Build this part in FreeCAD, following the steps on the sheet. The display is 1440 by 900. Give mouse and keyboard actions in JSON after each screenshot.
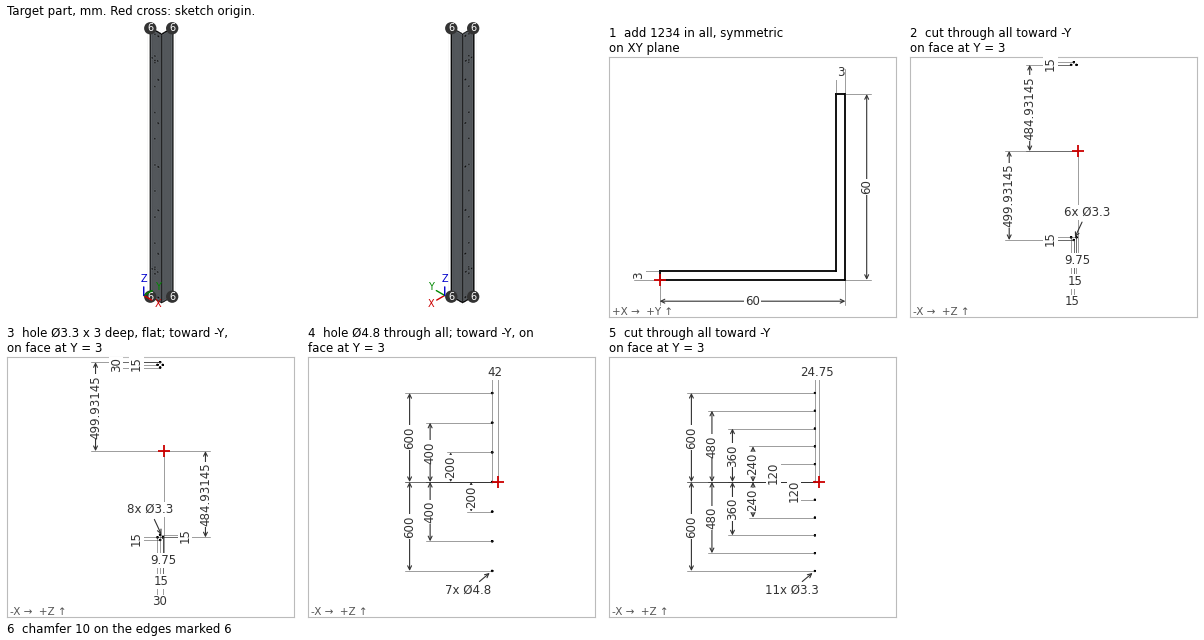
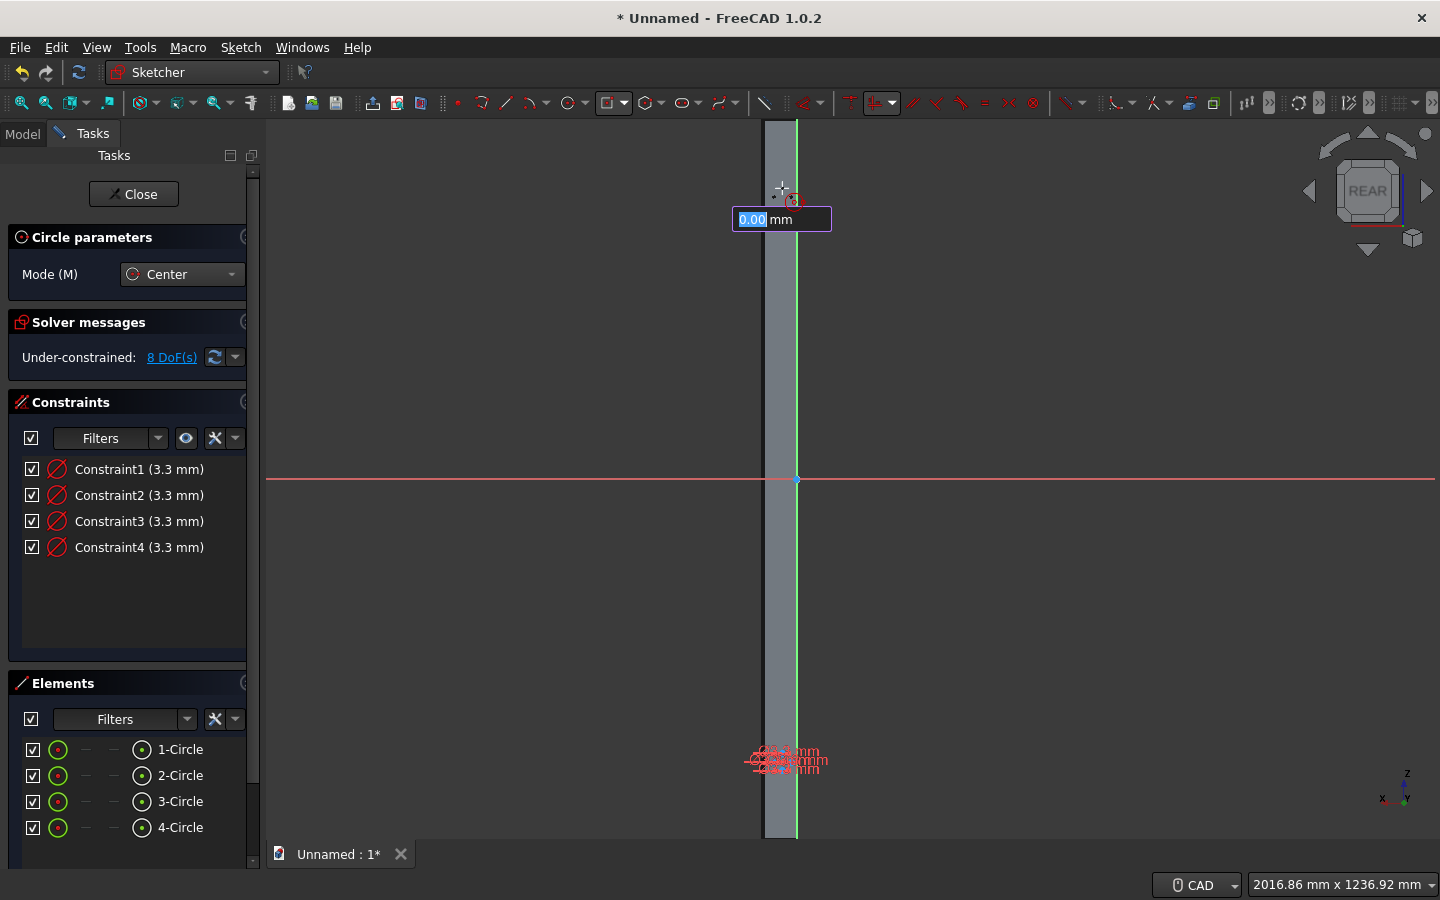
{"action": "type", "text": "3.3"}
{"action": "key", "text": "Return"}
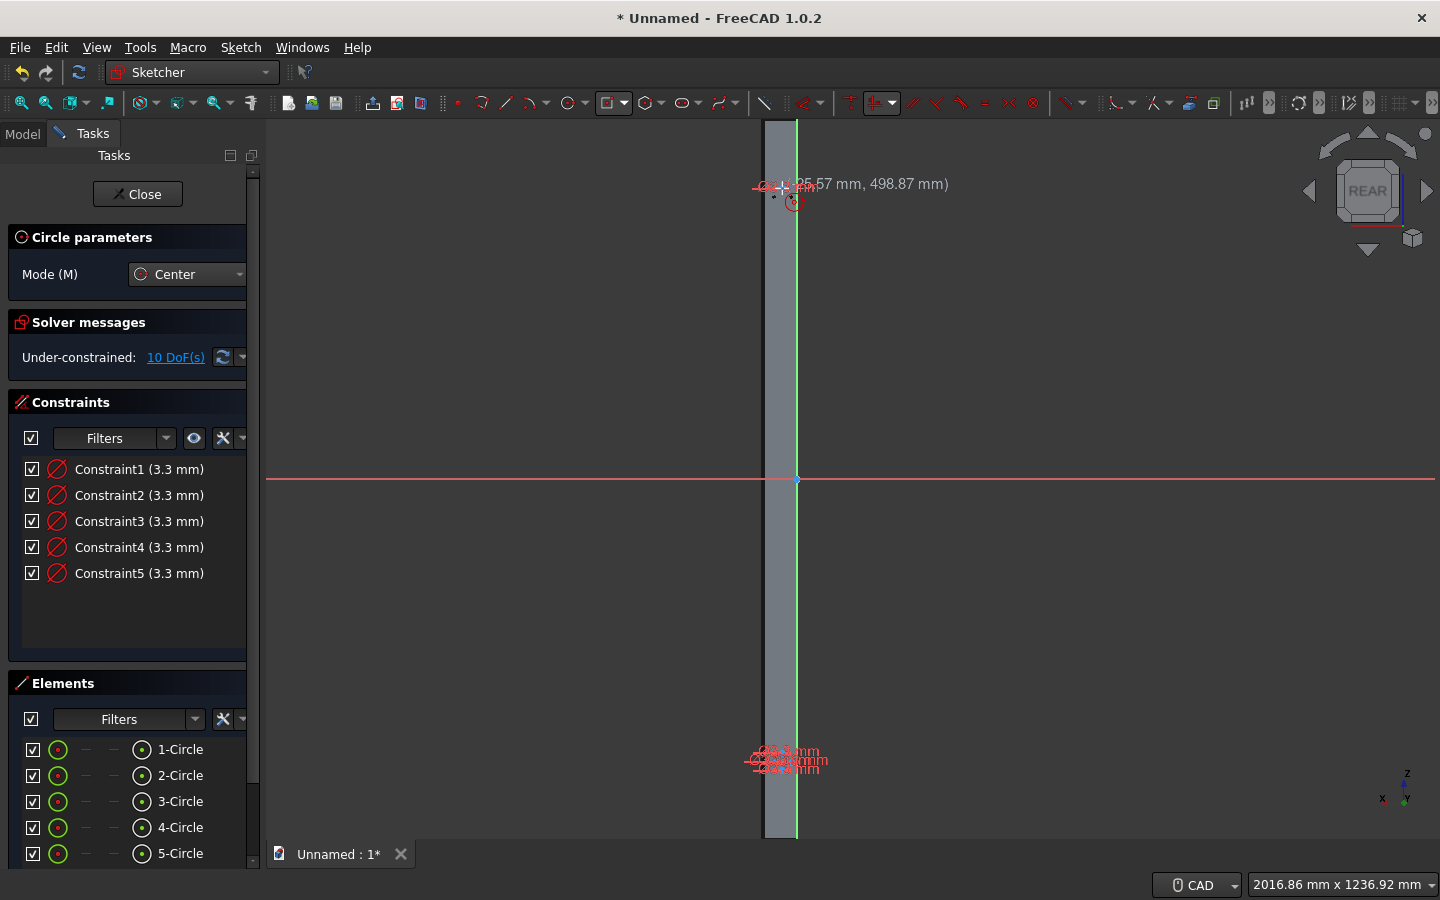
{"action": "scroll", "coordinate": [782, 206], "scroll_direction": "up", "scroll_amount": 16}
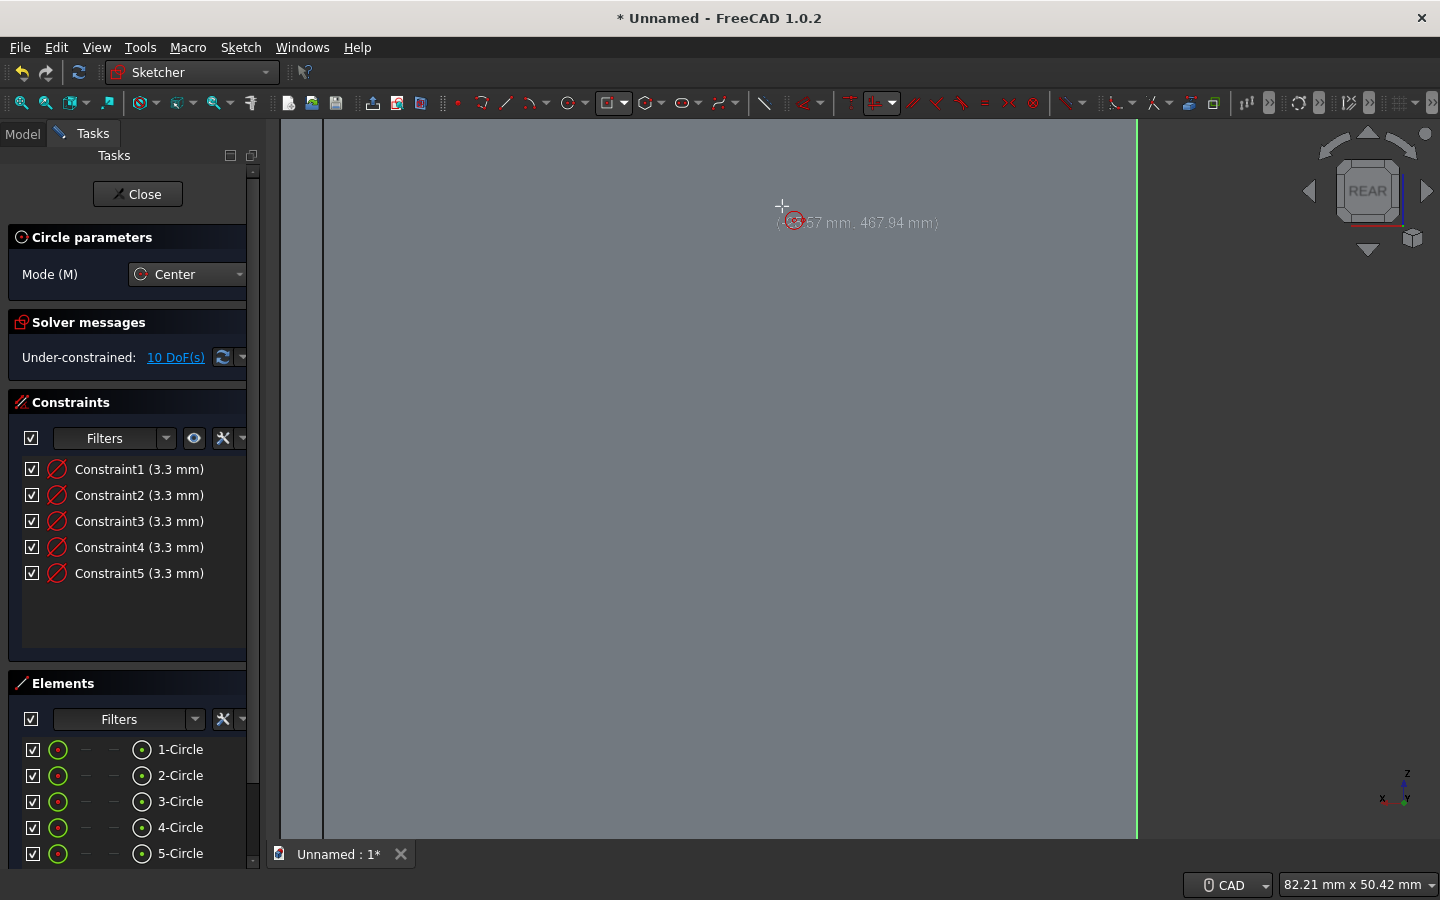
{"action": "scroll", "coordinate": [782, 206], "scroll_direction": "down", "scroll_amount": 16}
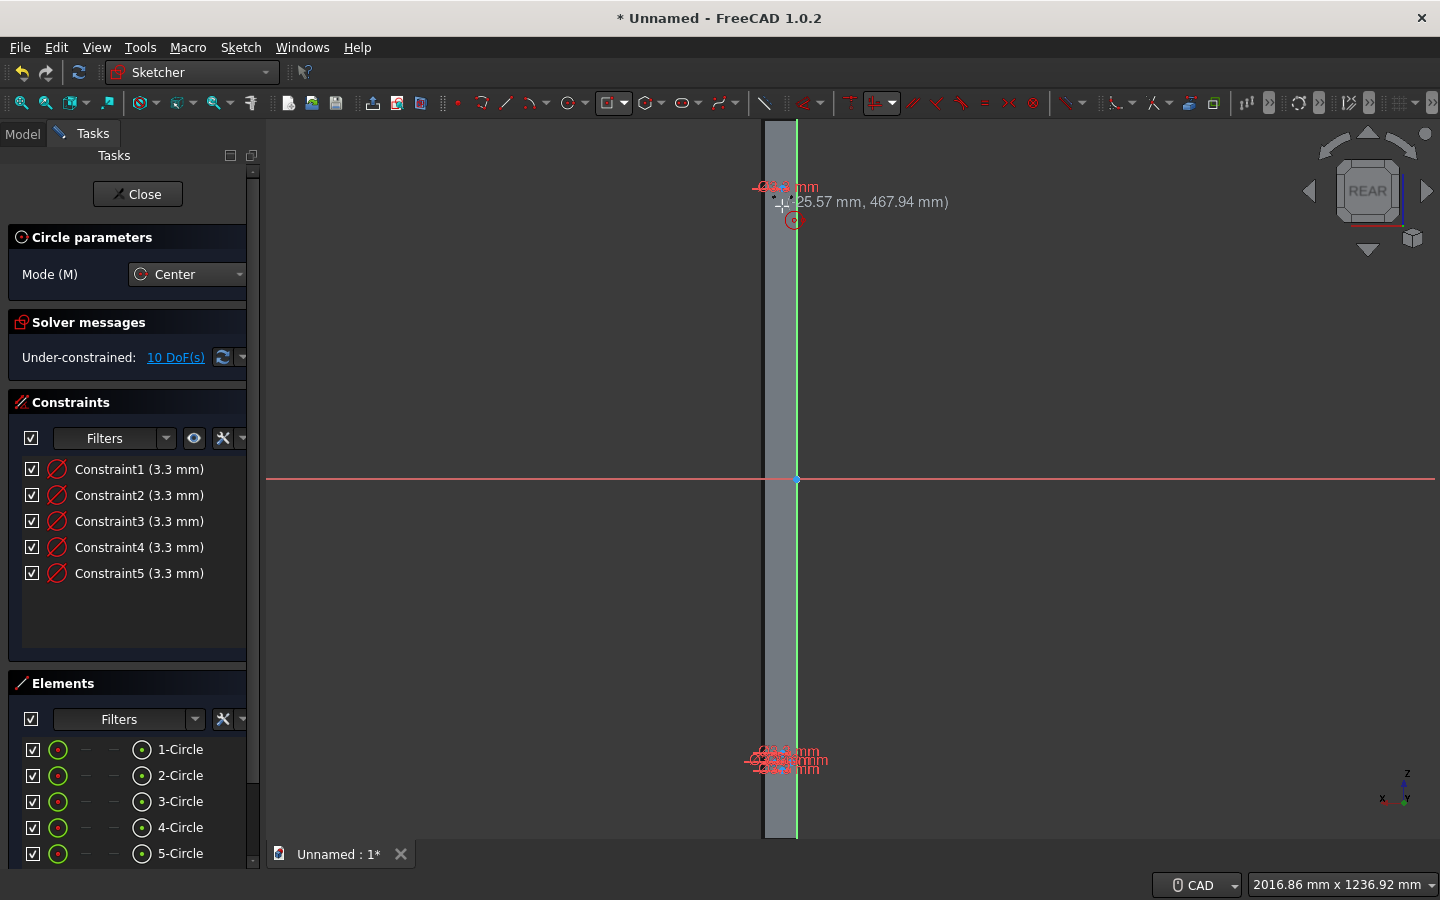
{"action": "left_click", "coordinate": [782, 206]}
{"action": "mouse_move", "coordinate": [782, 205]}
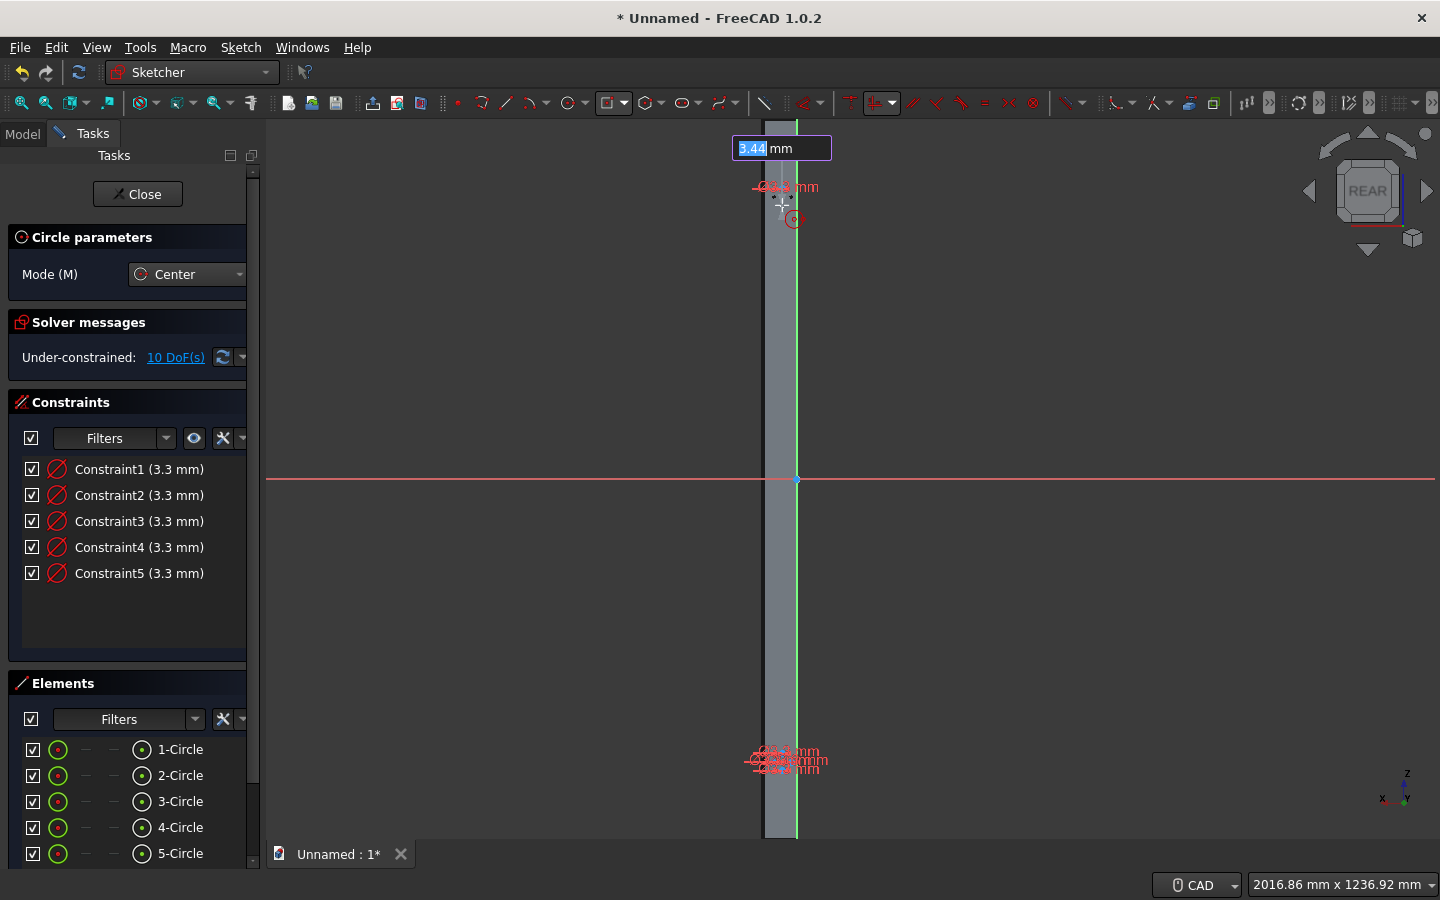
{"action": "type", "text": "3.3"}
{"action": "key", "text": "Return"}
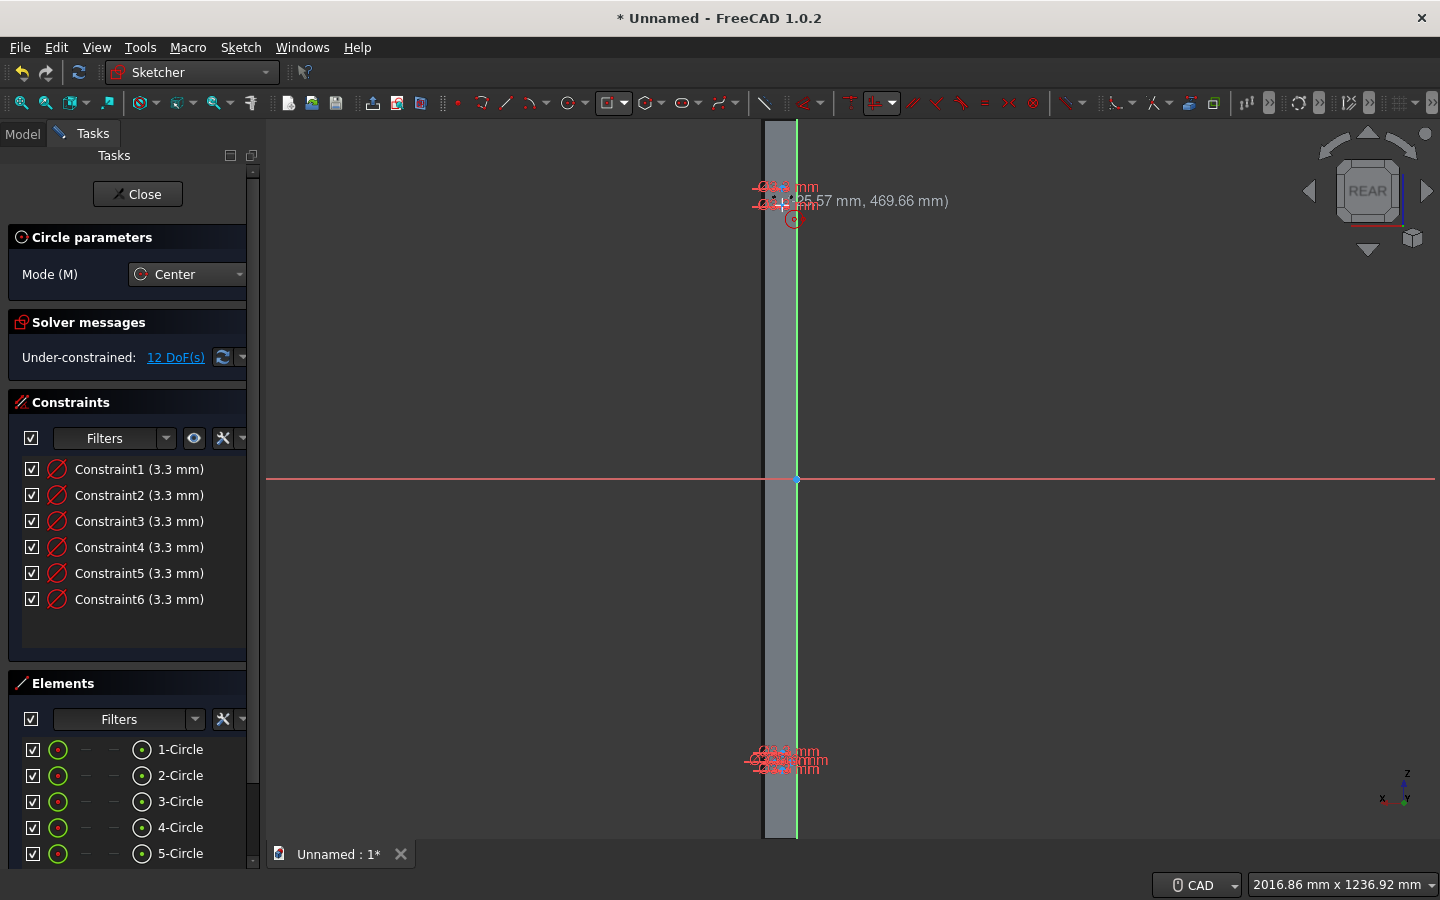
{"action": "scroll", "coordinate": [774, 197], "scroll_direction": "up", "scroll_amount": 16}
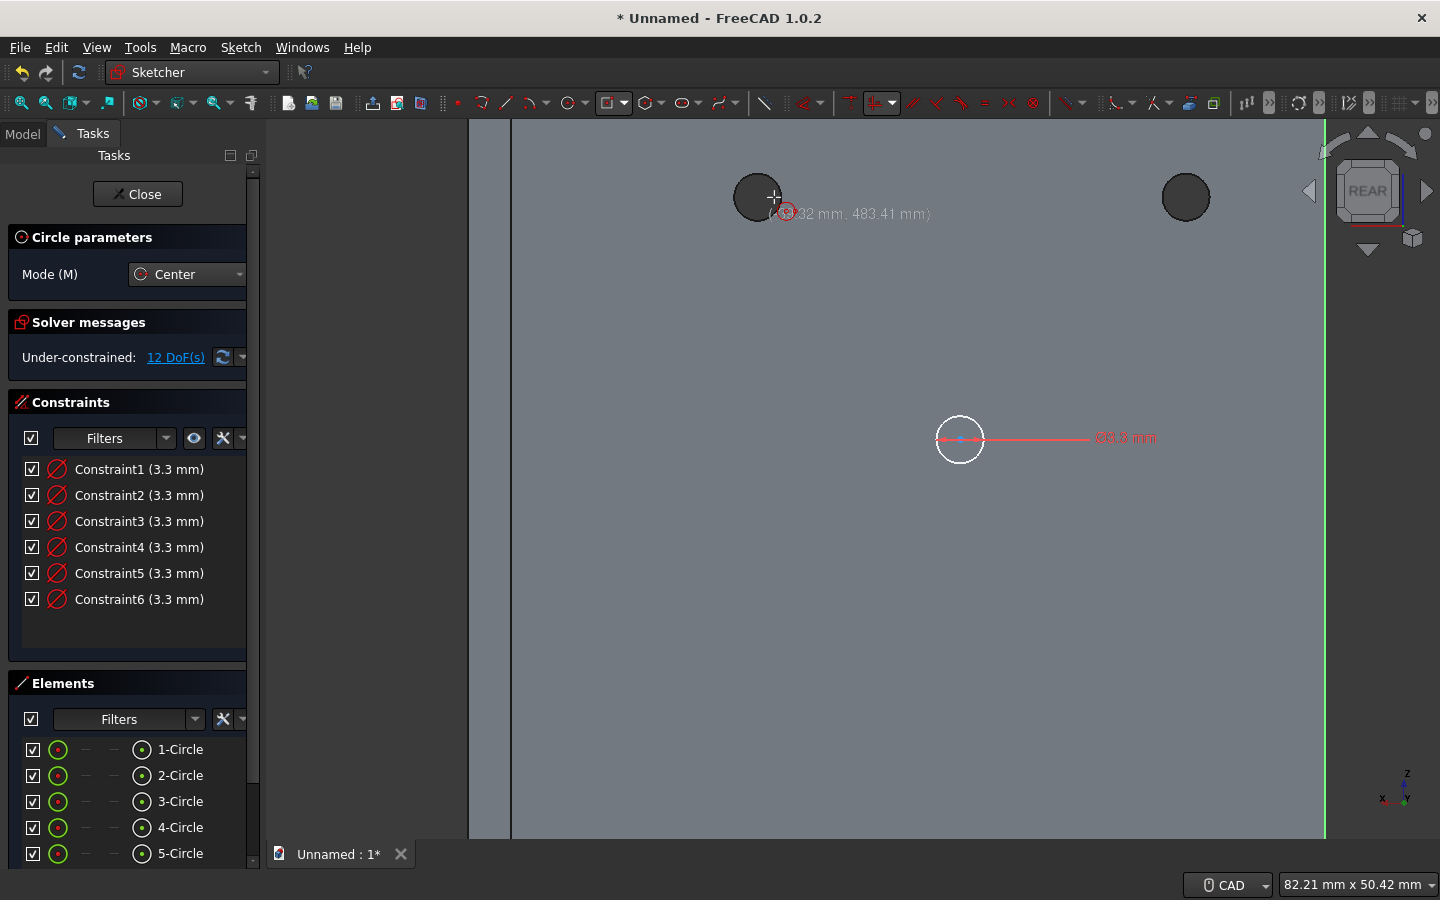
{"action": "scroll", "coordinate": [774, 197], "scroll_direction": "down", "scroll_amount": 16}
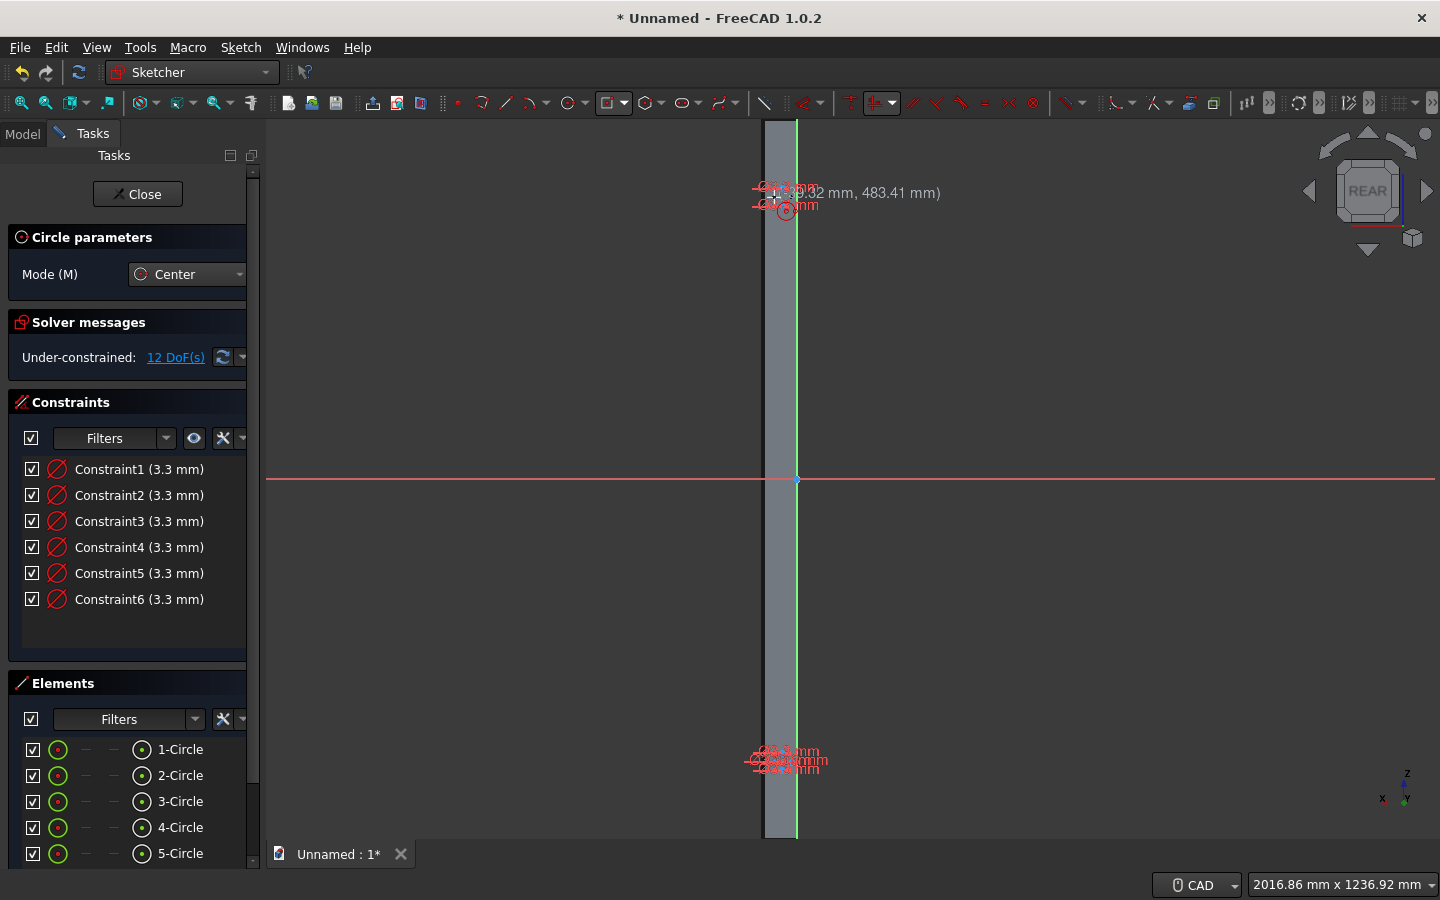
{"action": "scroll", "coordinate": [774, 197], "scroll_direction": "up", "scroll_amount": 2}